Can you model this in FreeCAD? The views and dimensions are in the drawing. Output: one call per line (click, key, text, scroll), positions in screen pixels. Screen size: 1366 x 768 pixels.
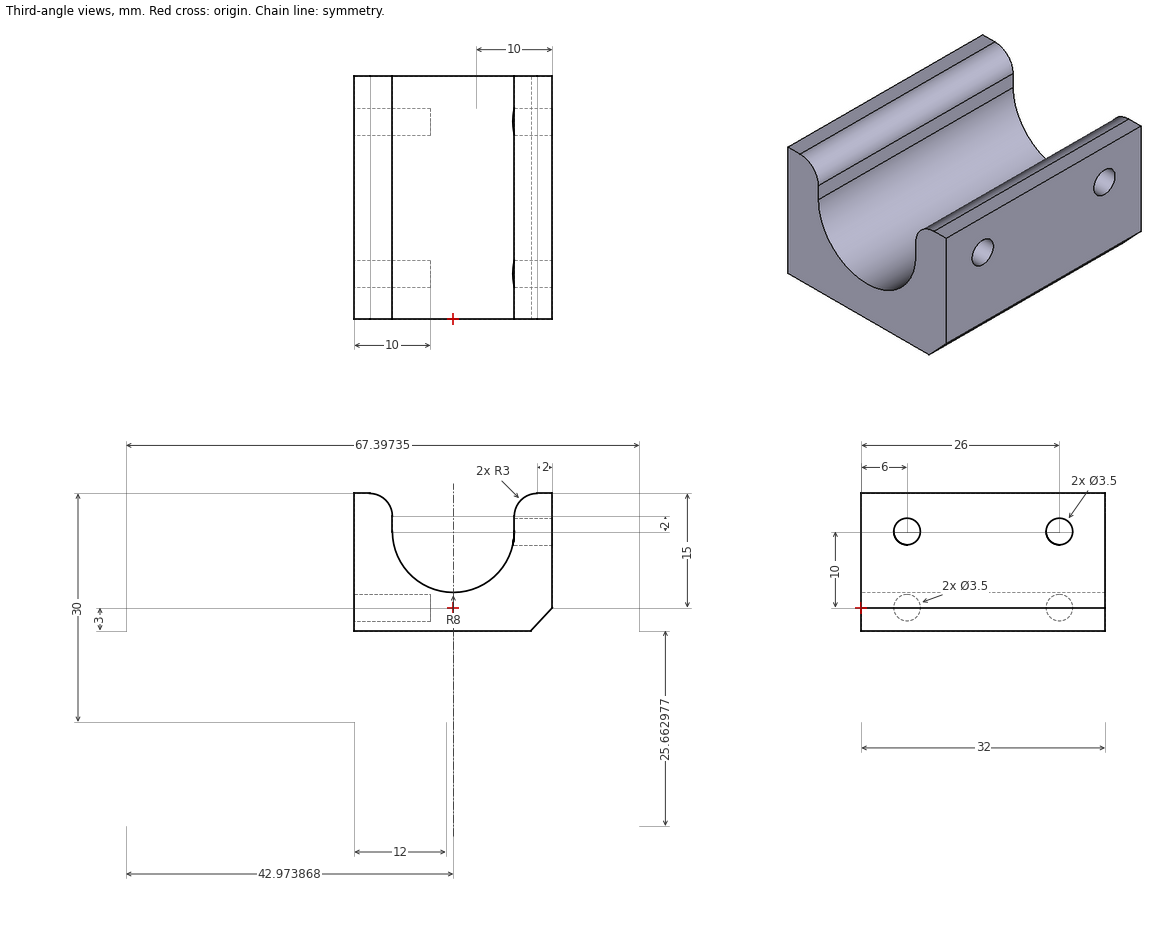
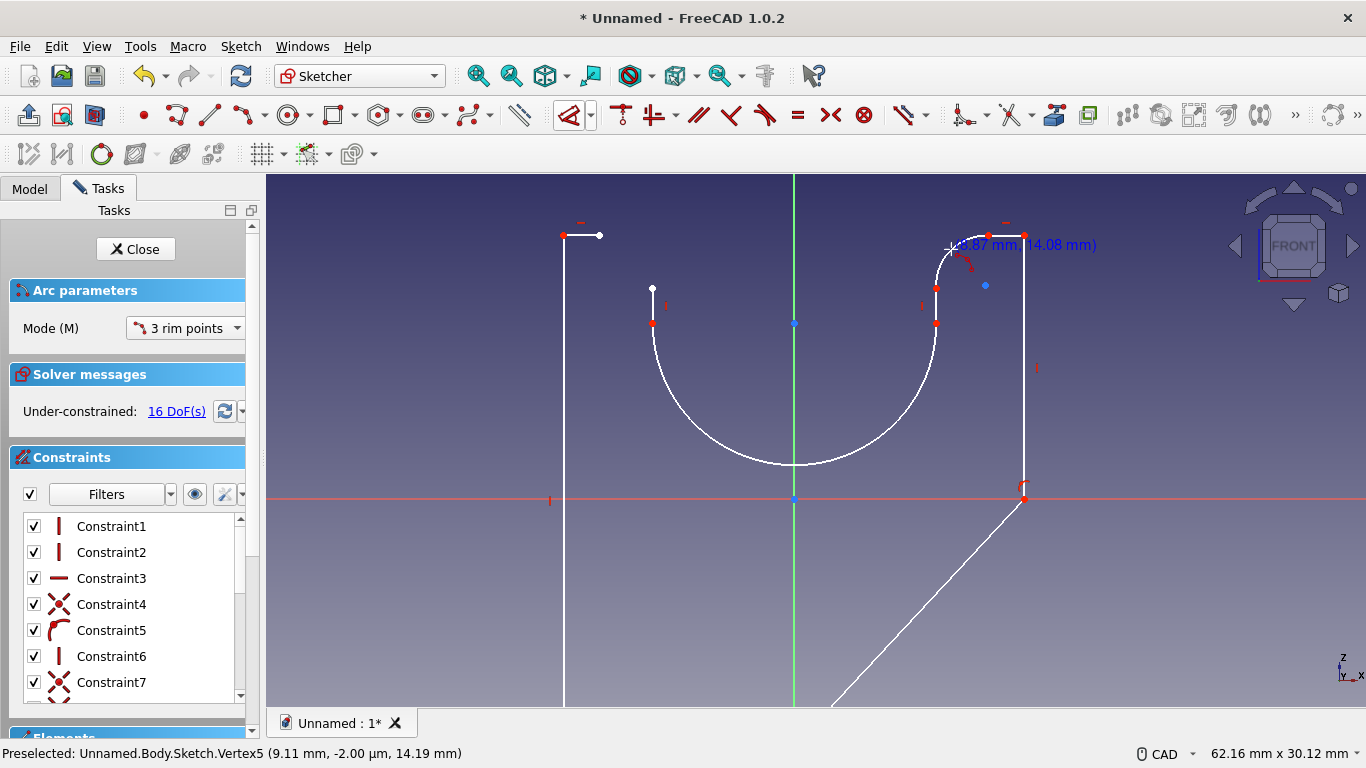
click(599, 235)
click(653, 288)
click(637, 249)
key(Escape)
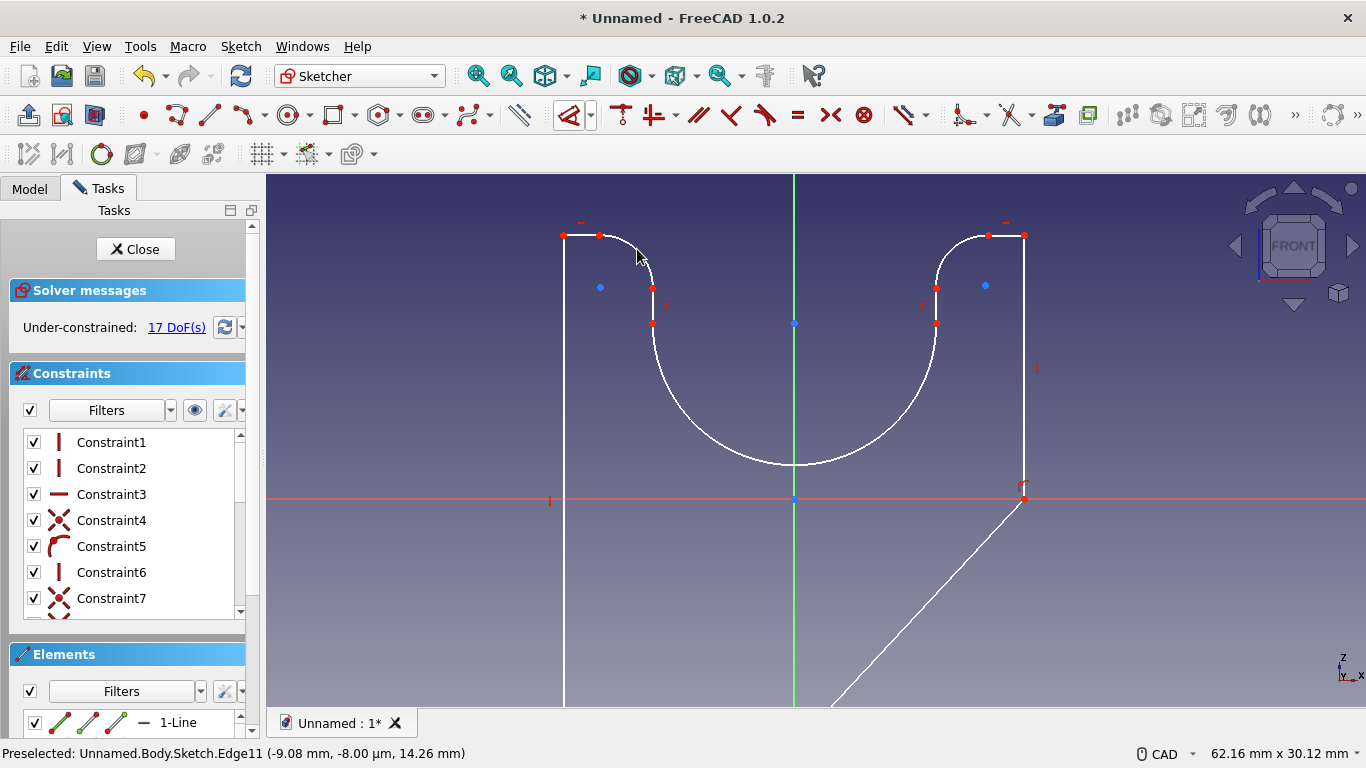
scroll(653, 299, up, 2)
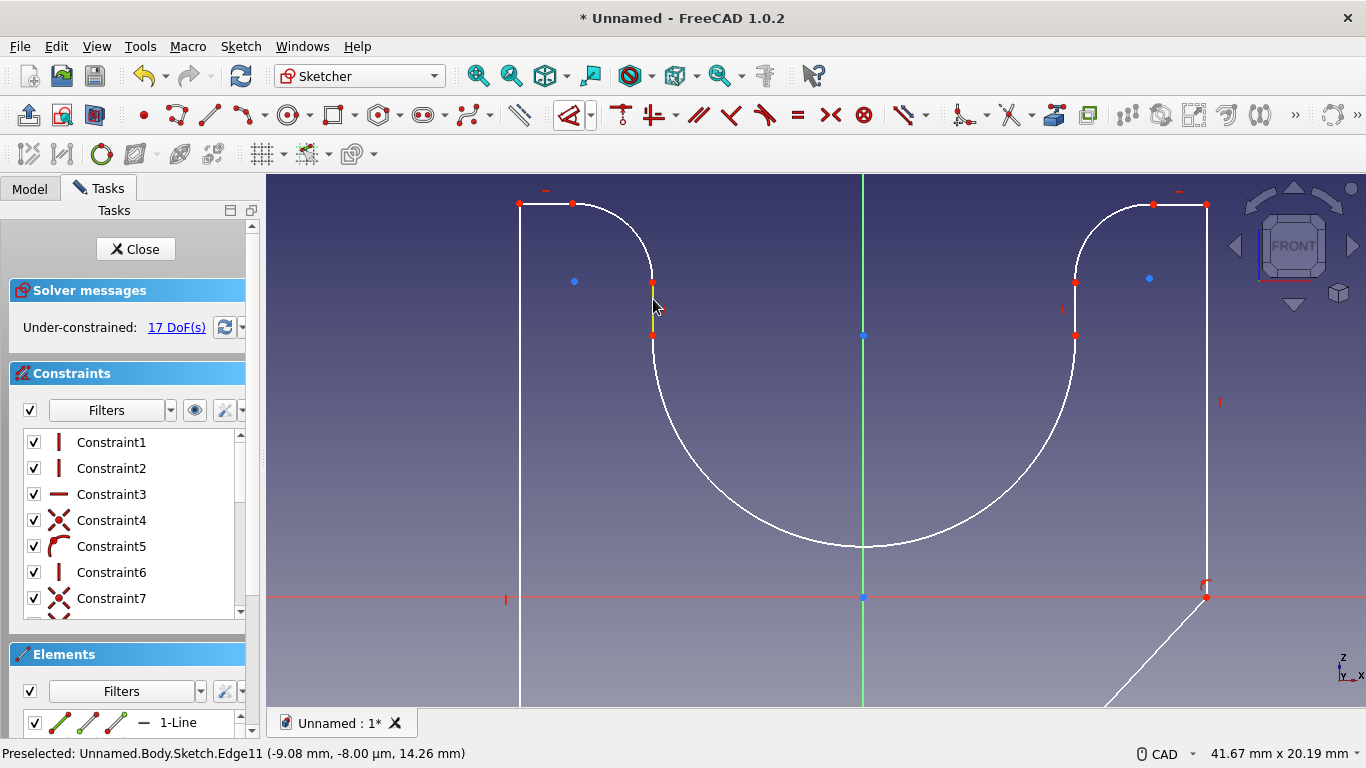
click(653, 299)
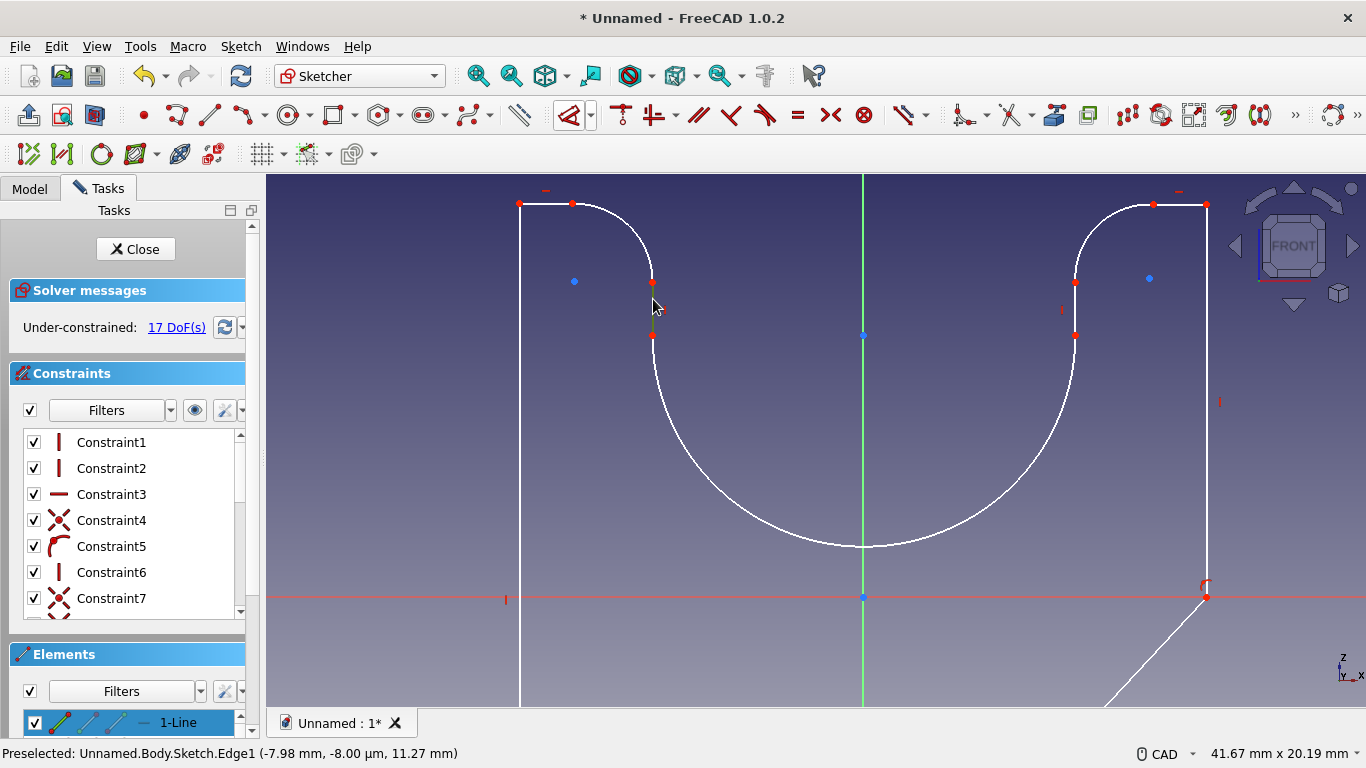
click(740, 507)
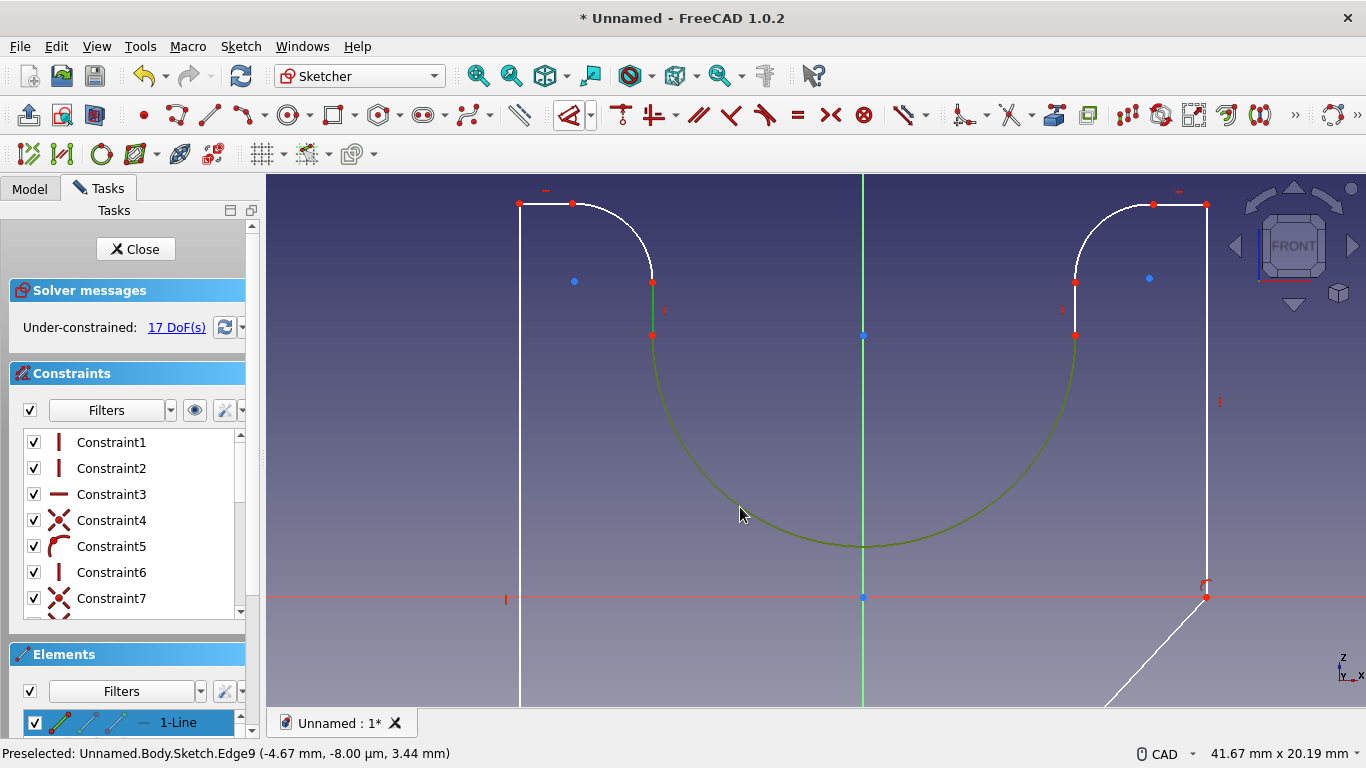
click(765, 116)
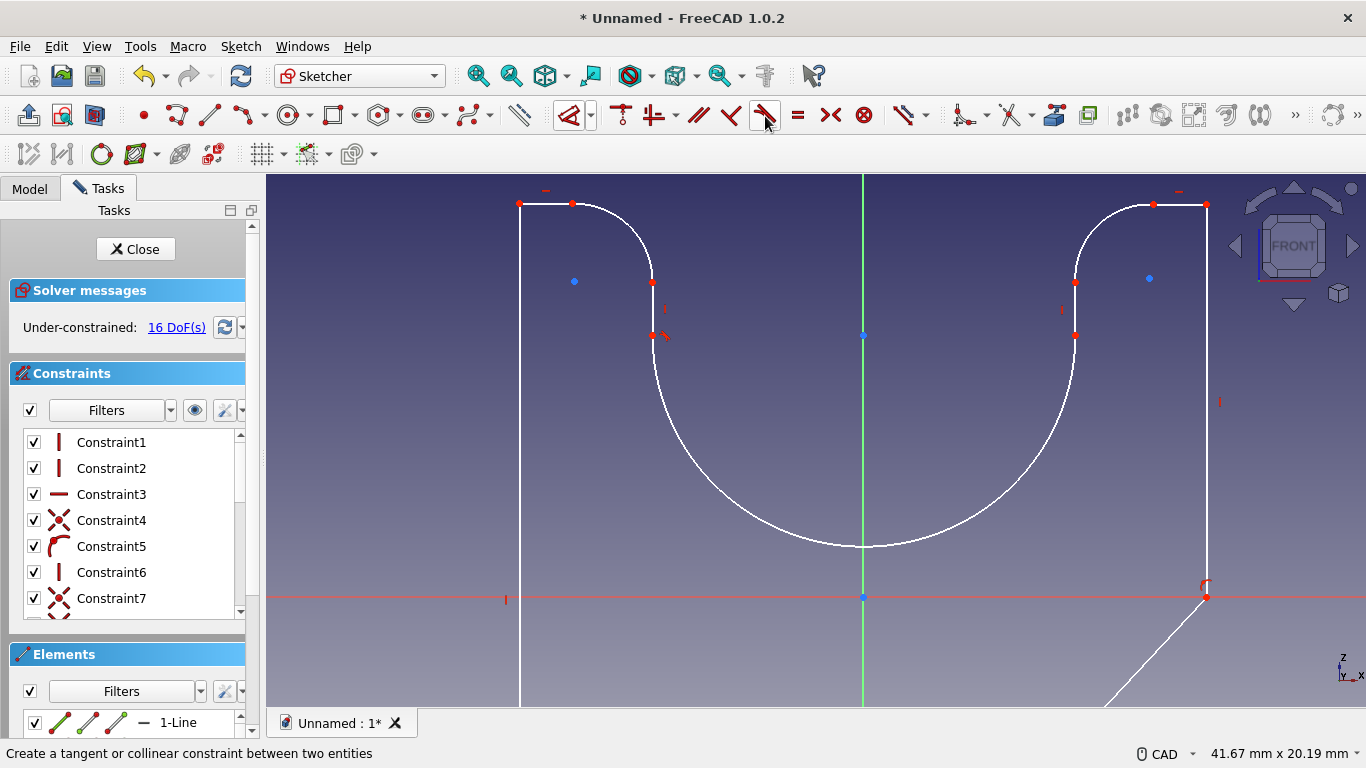
click(653, 298)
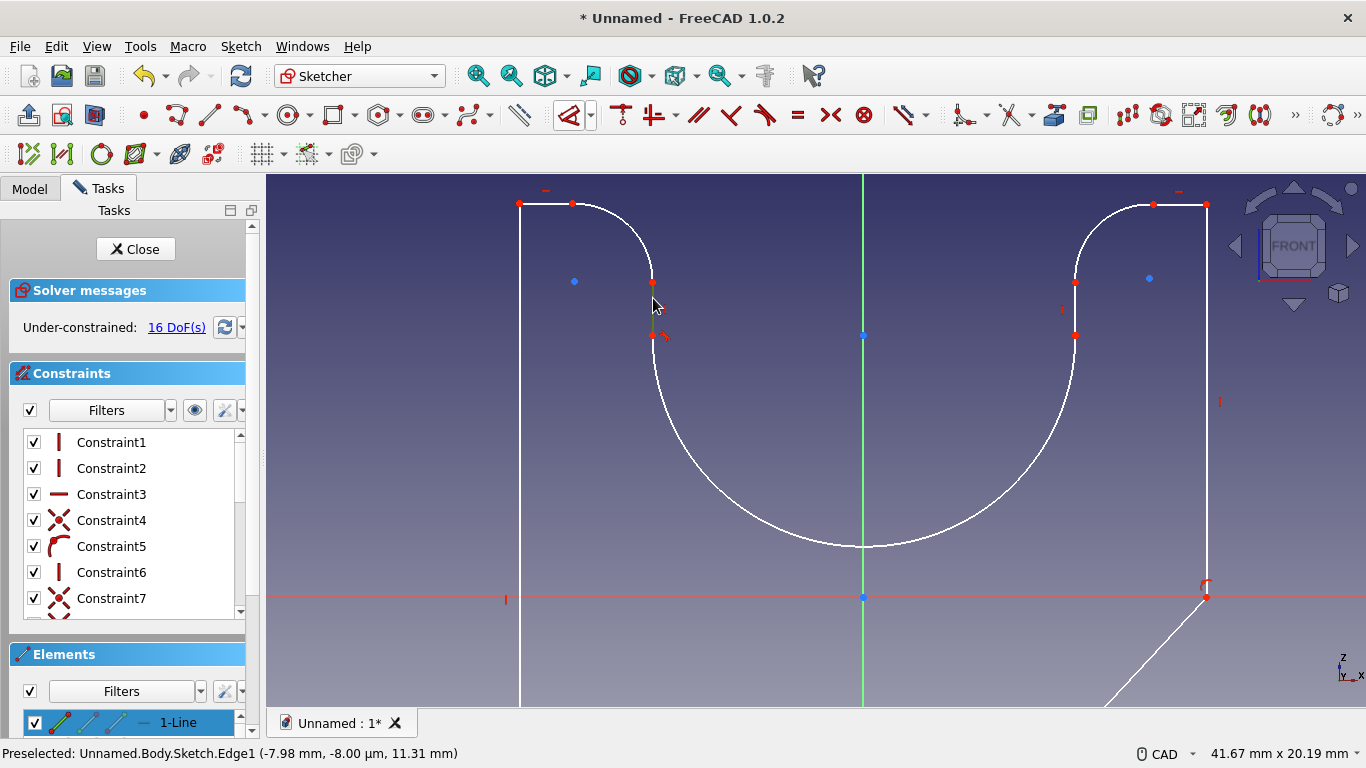
click(644, 246)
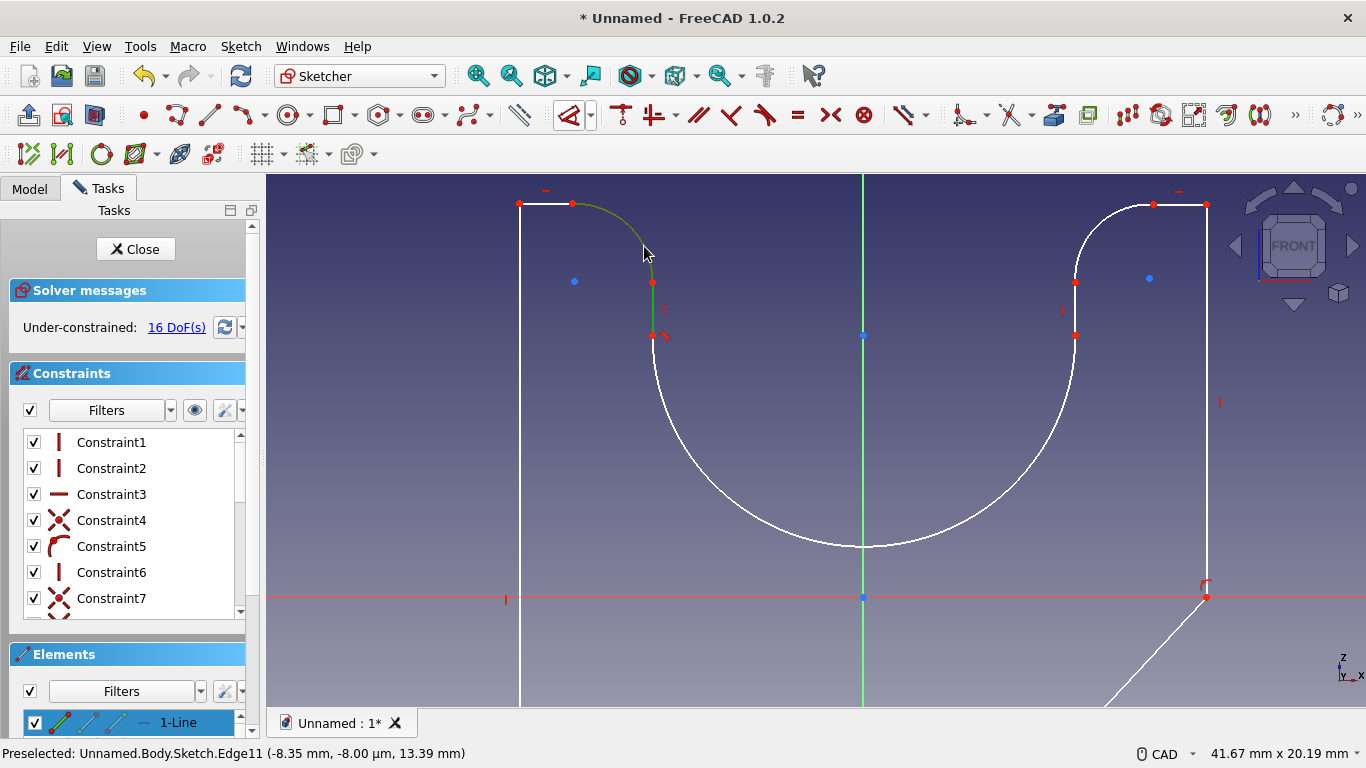
click(765, 116)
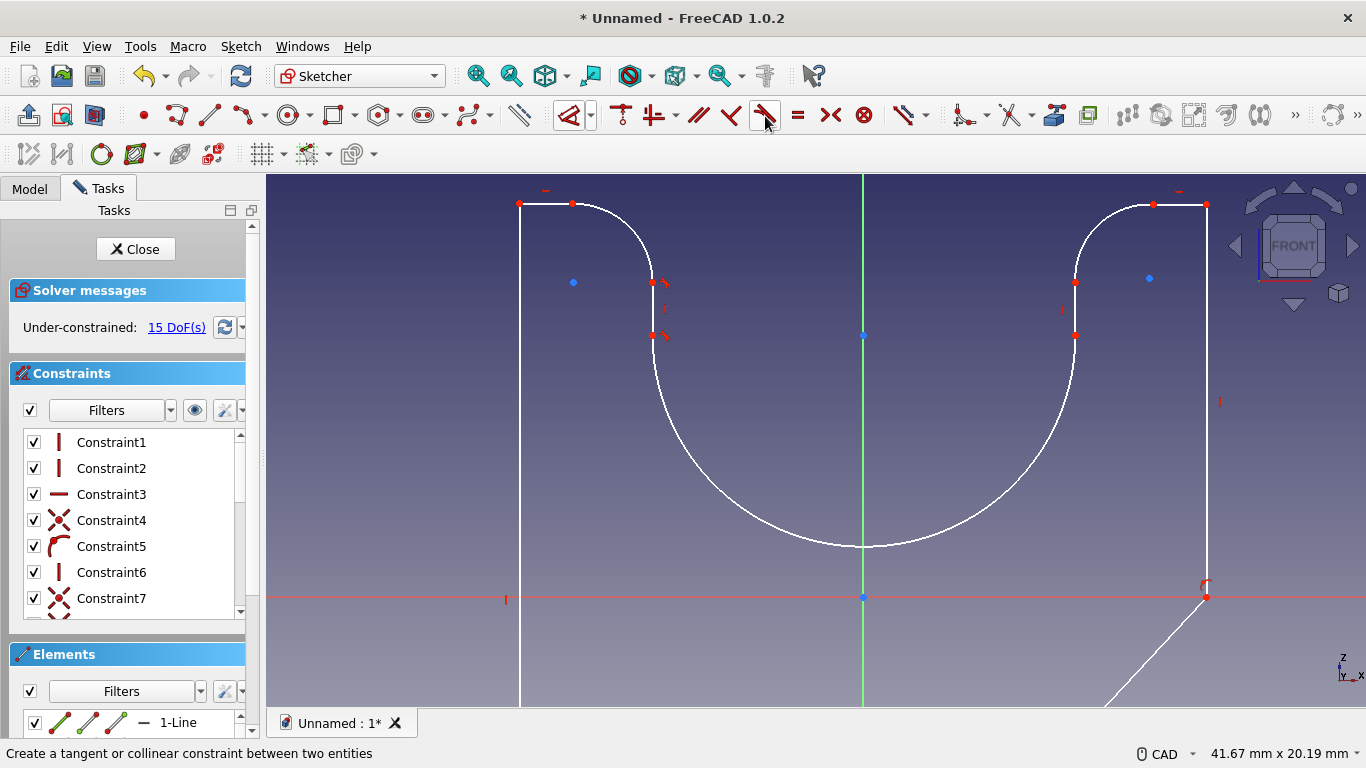
click(1075, 320)